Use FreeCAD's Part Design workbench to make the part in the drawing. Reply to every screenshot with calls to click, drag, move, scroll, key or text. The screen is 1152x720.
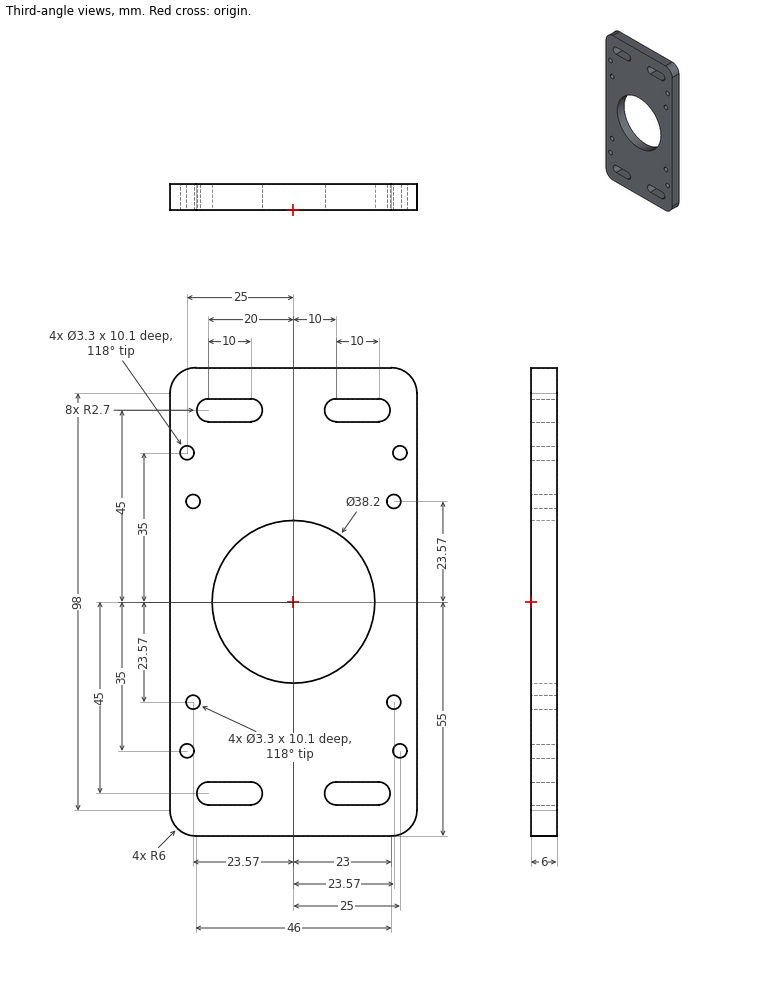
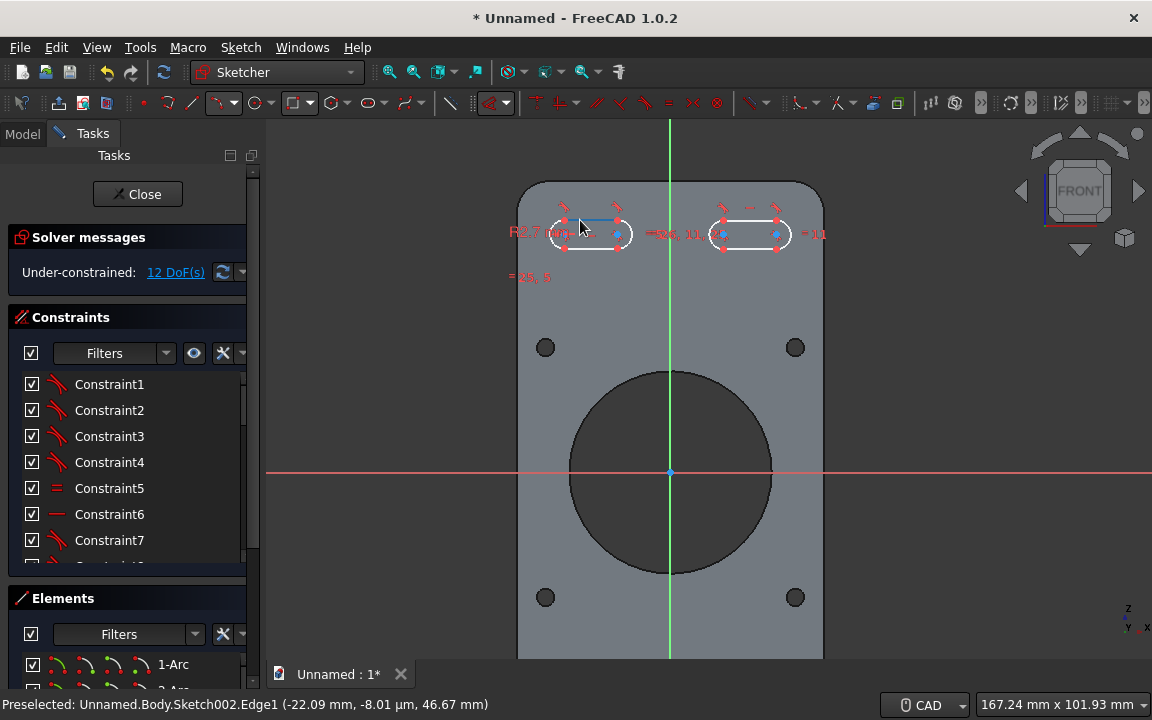
click(580, 220)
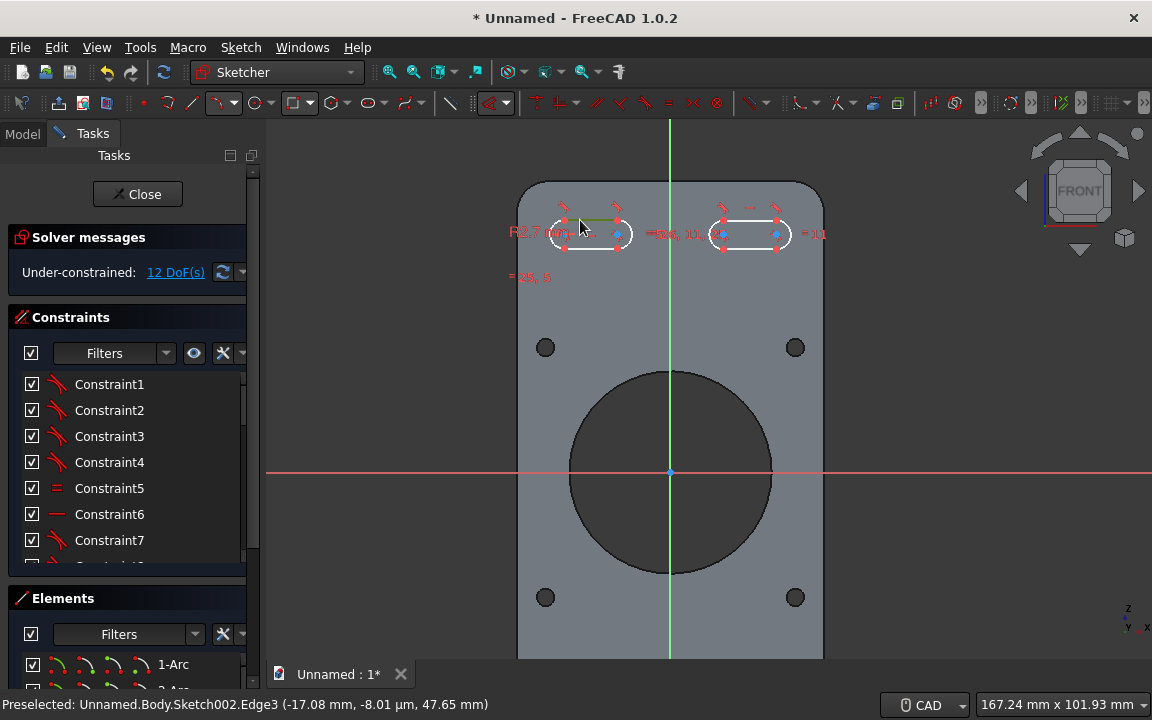
key(l)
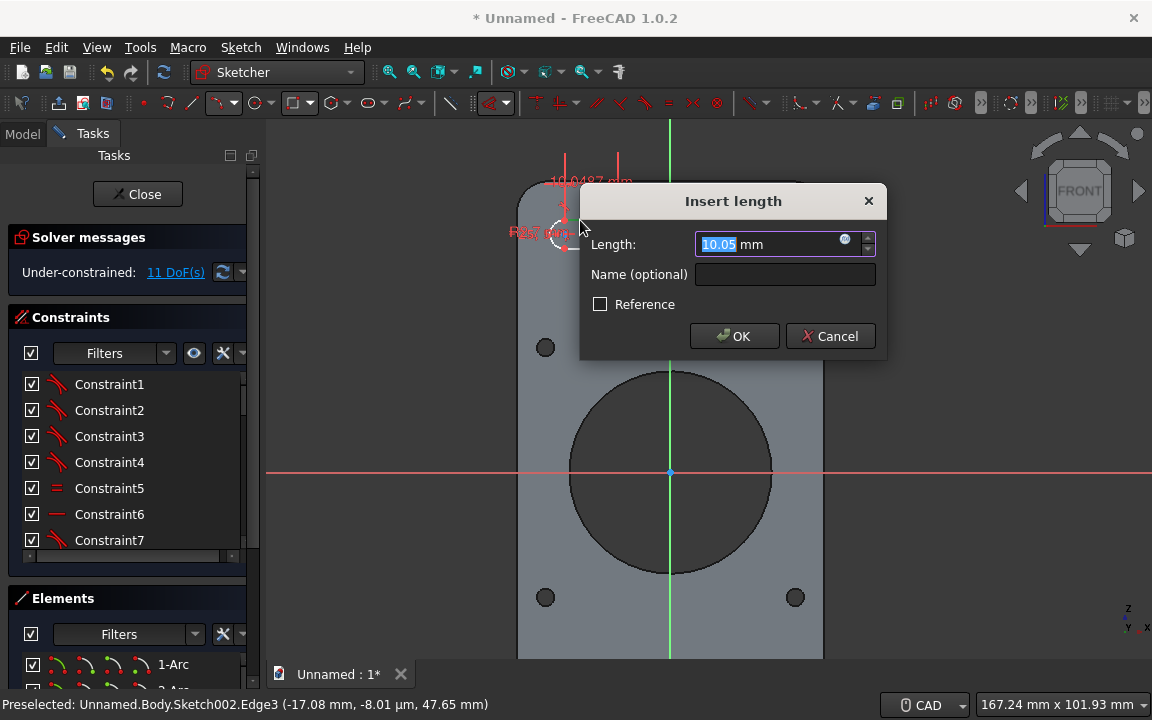
text(10)
key(Return)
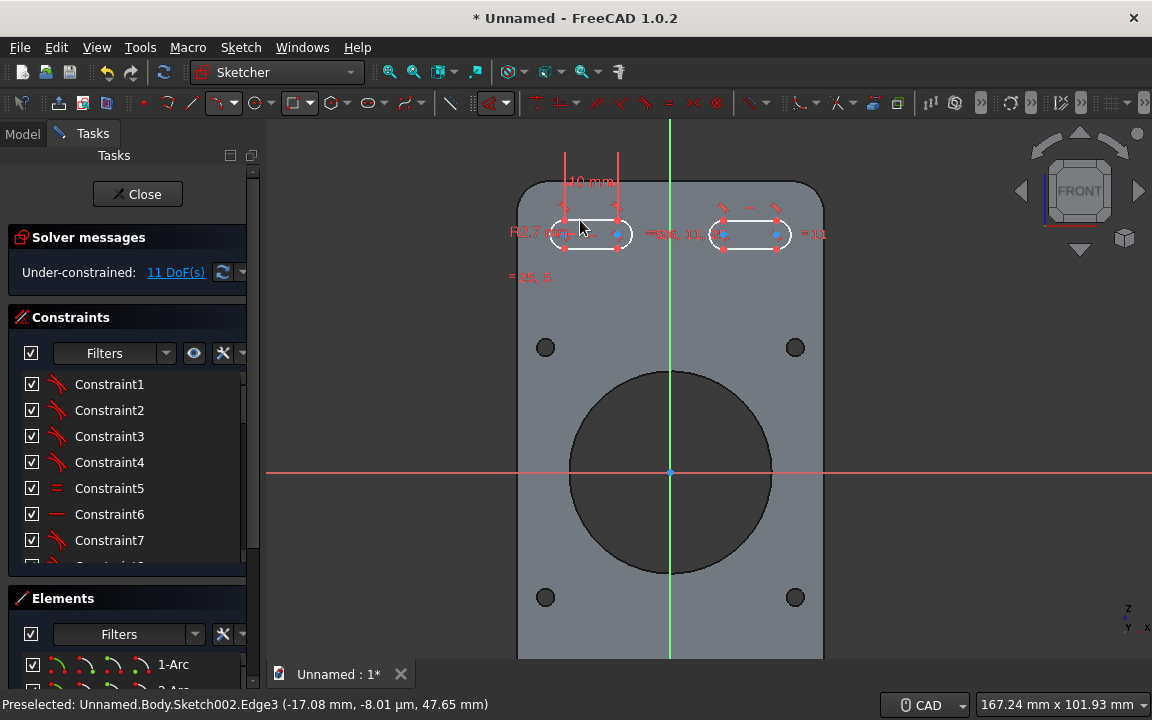
click(740, 221)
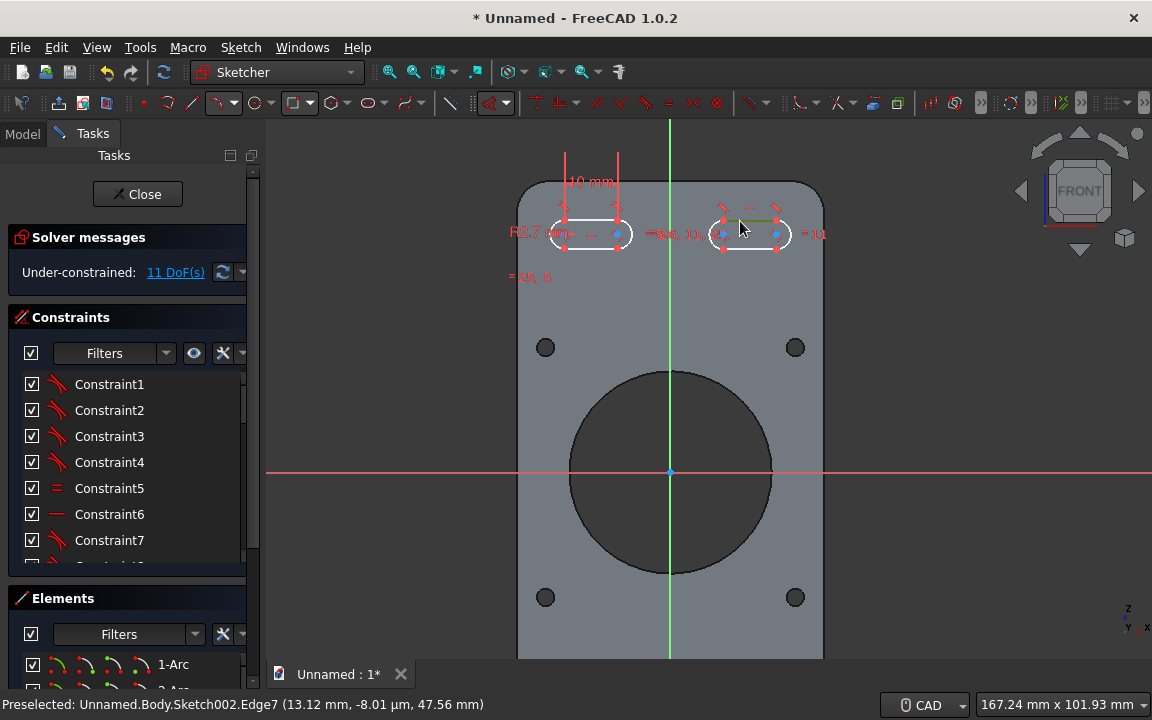
key(l)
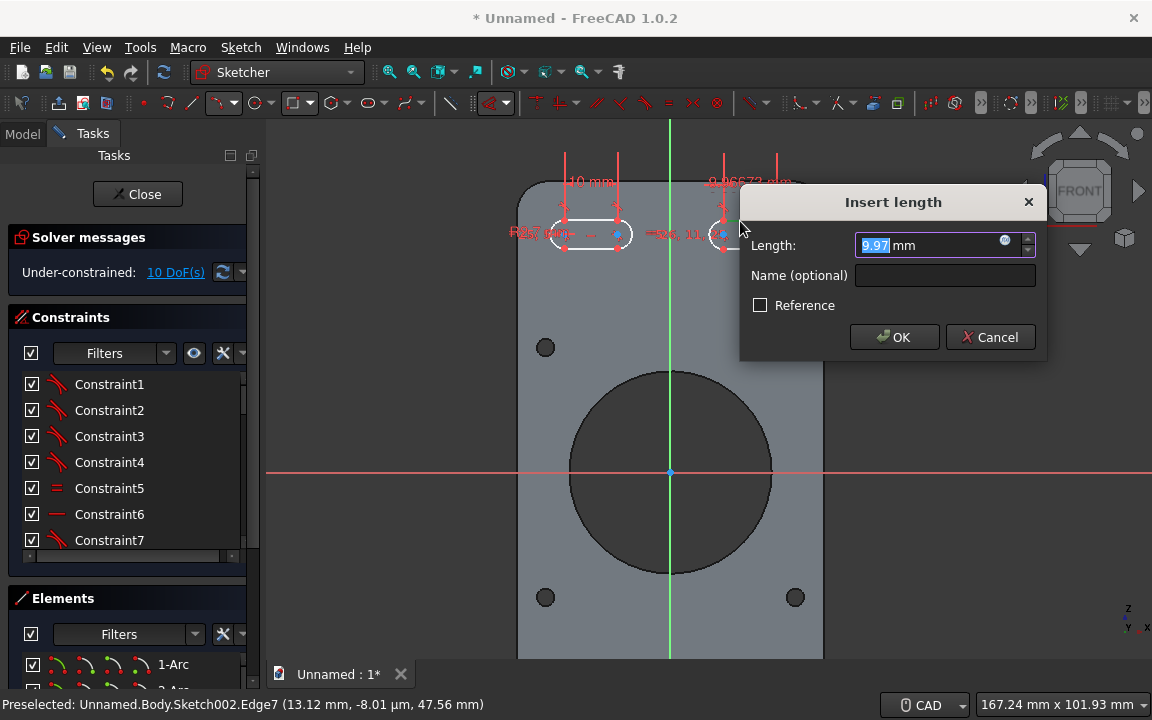
text(10)
key(Return)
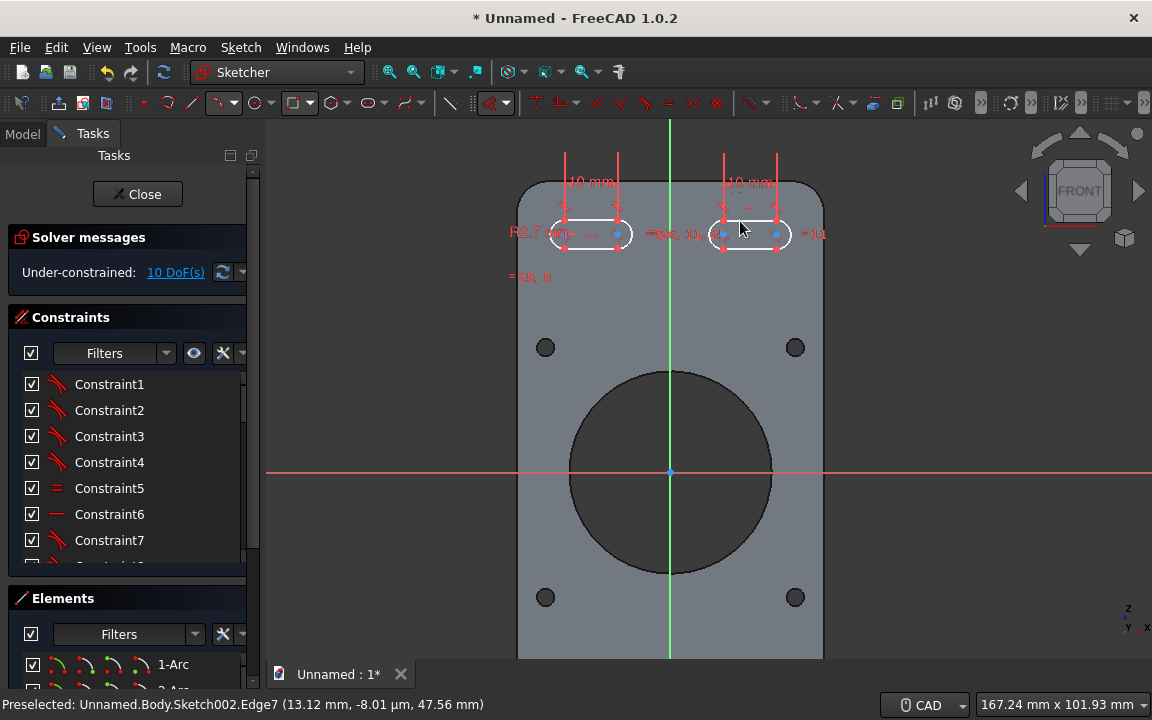
scroll(580, 219, down, 2)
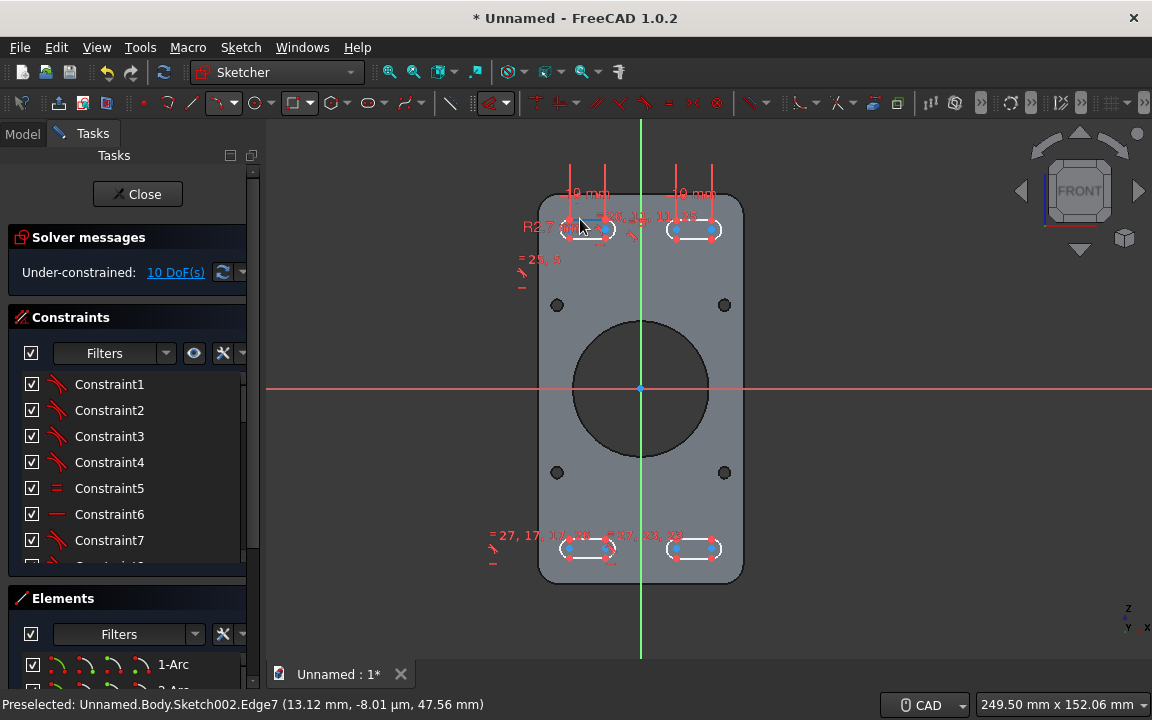
scroll(580, 539, up, 2)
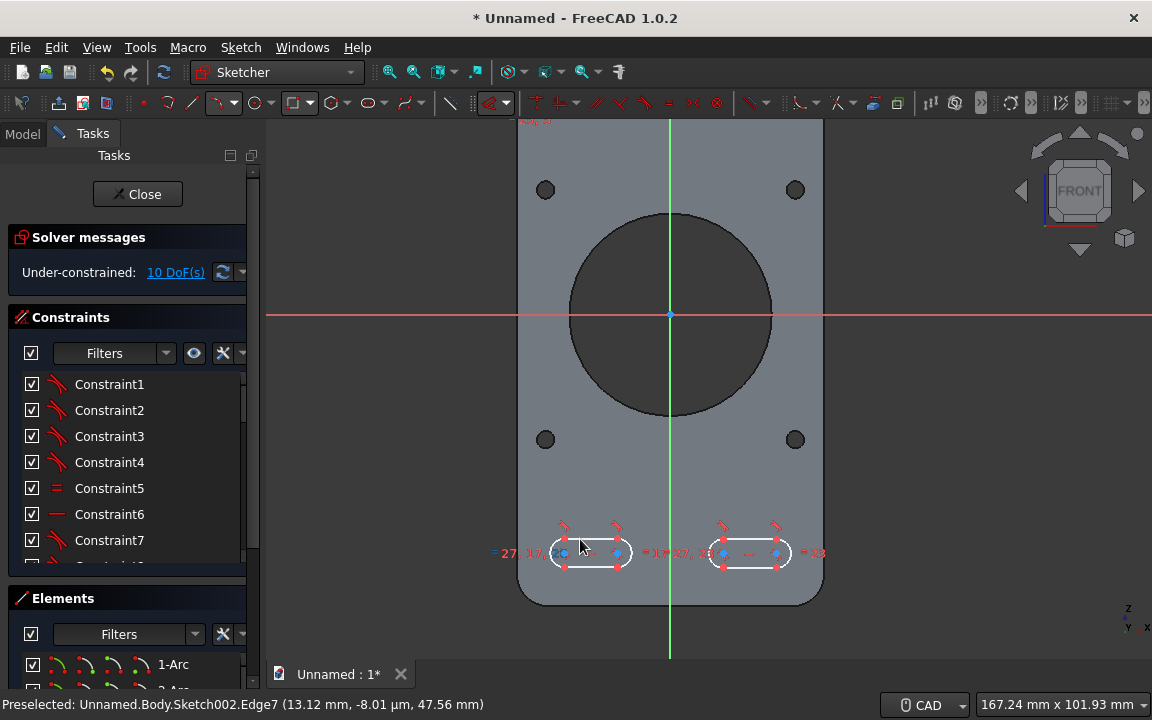
click(580, 539)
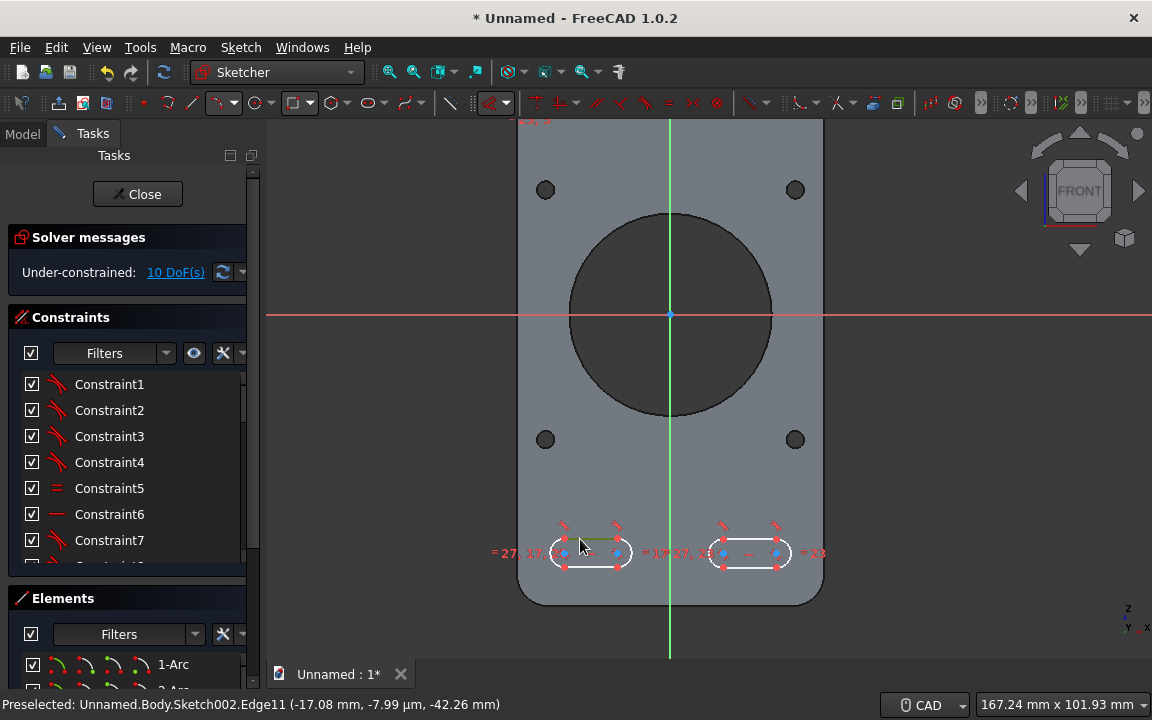
key(l)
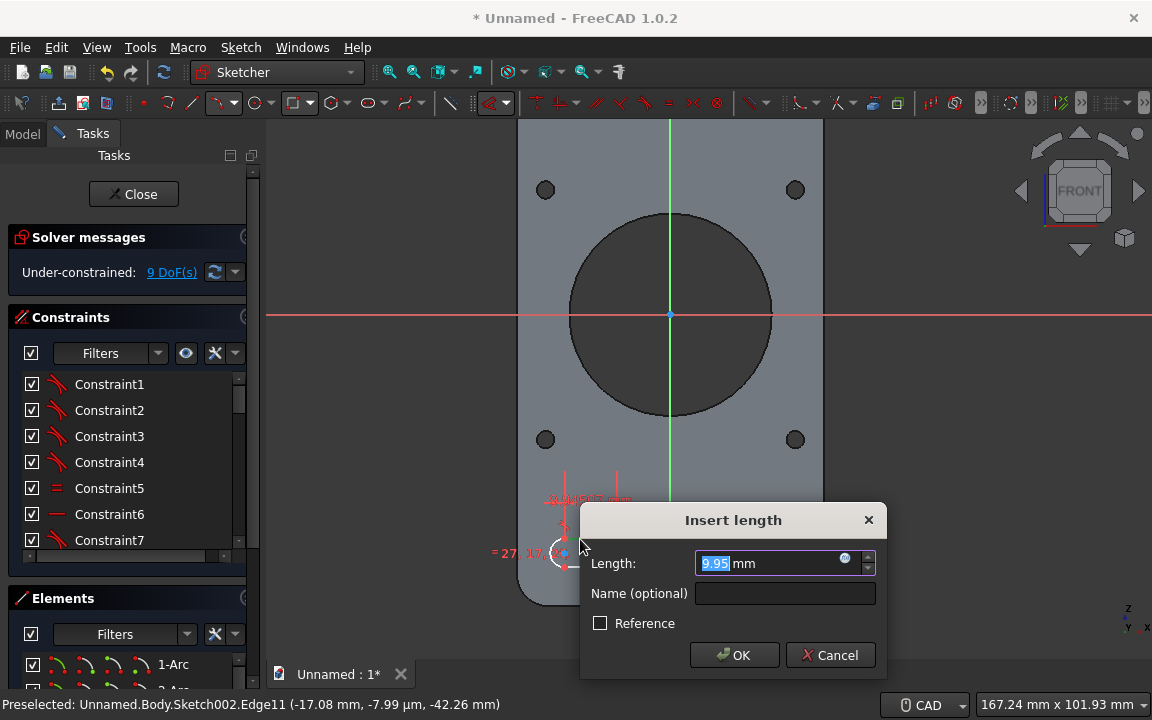
text(10)
key(Return)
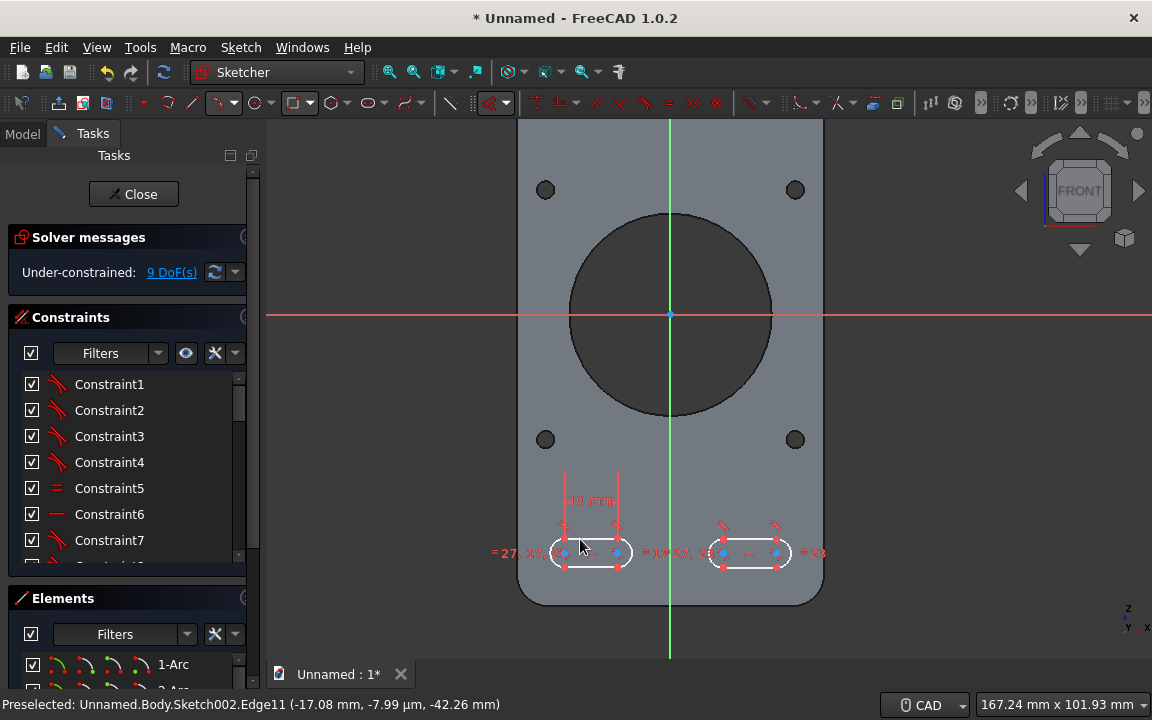
click(739, 539)